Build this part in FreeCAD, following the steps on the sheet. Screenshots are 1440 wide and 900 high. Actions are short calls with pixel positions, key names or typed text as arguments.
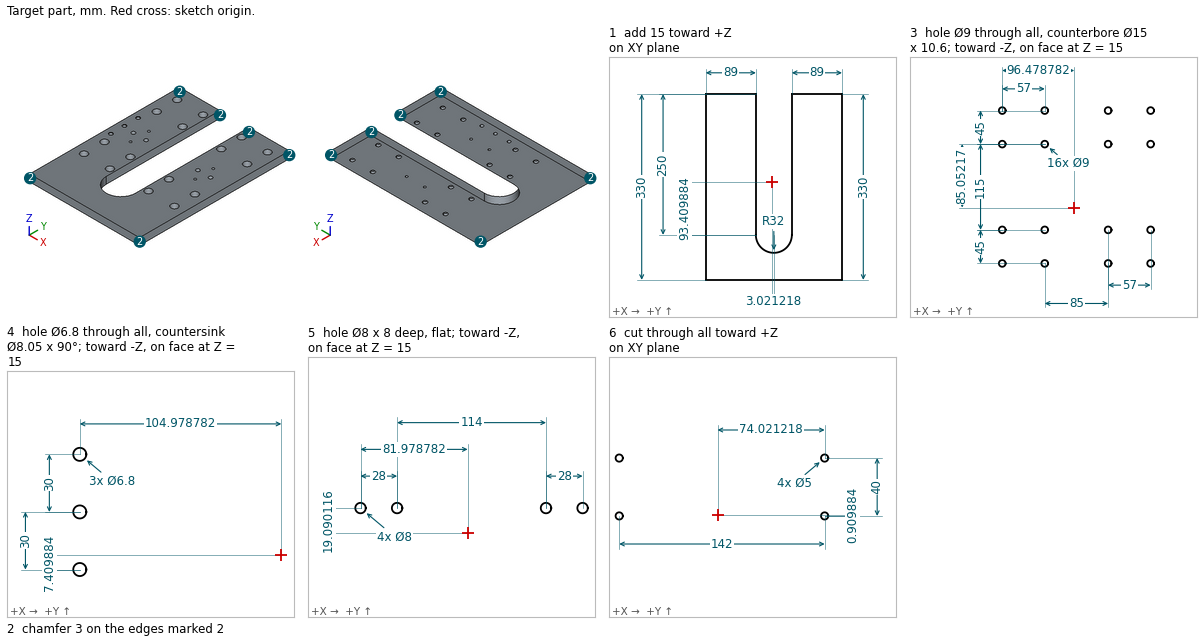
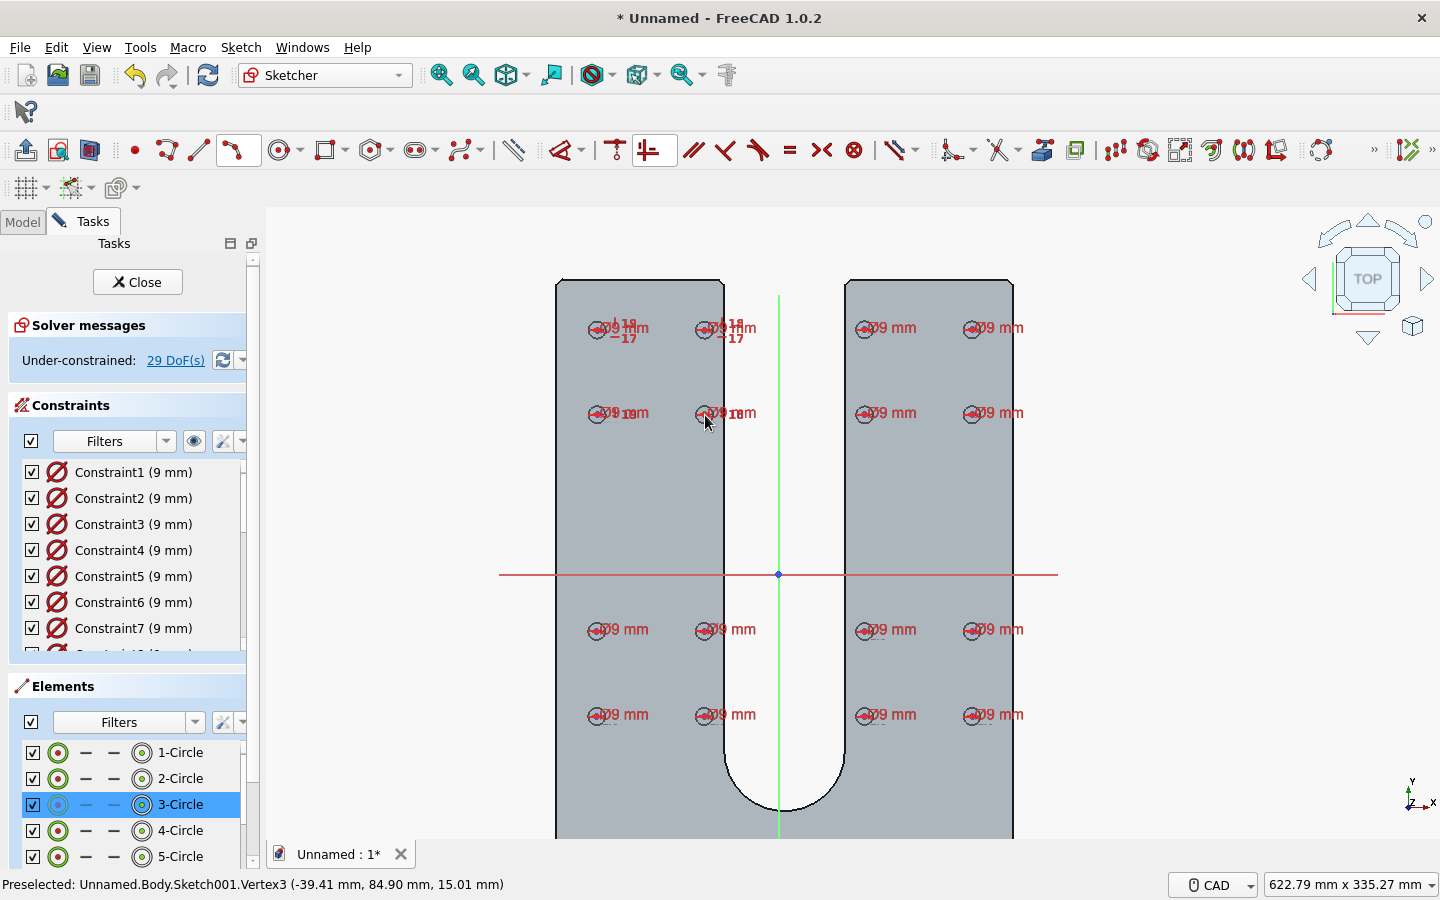
click(597, 415)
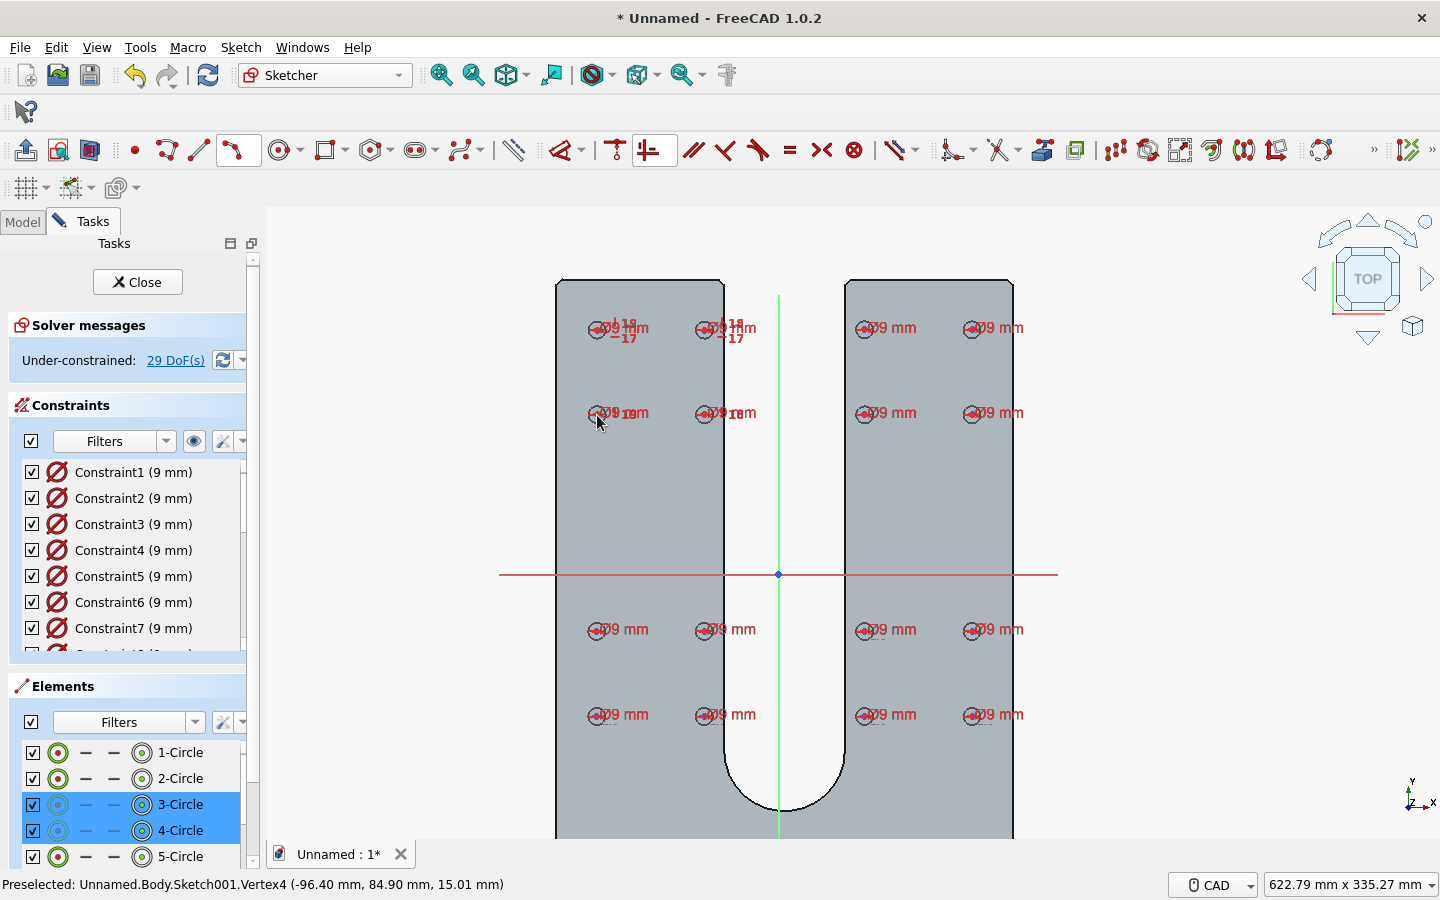
key(h)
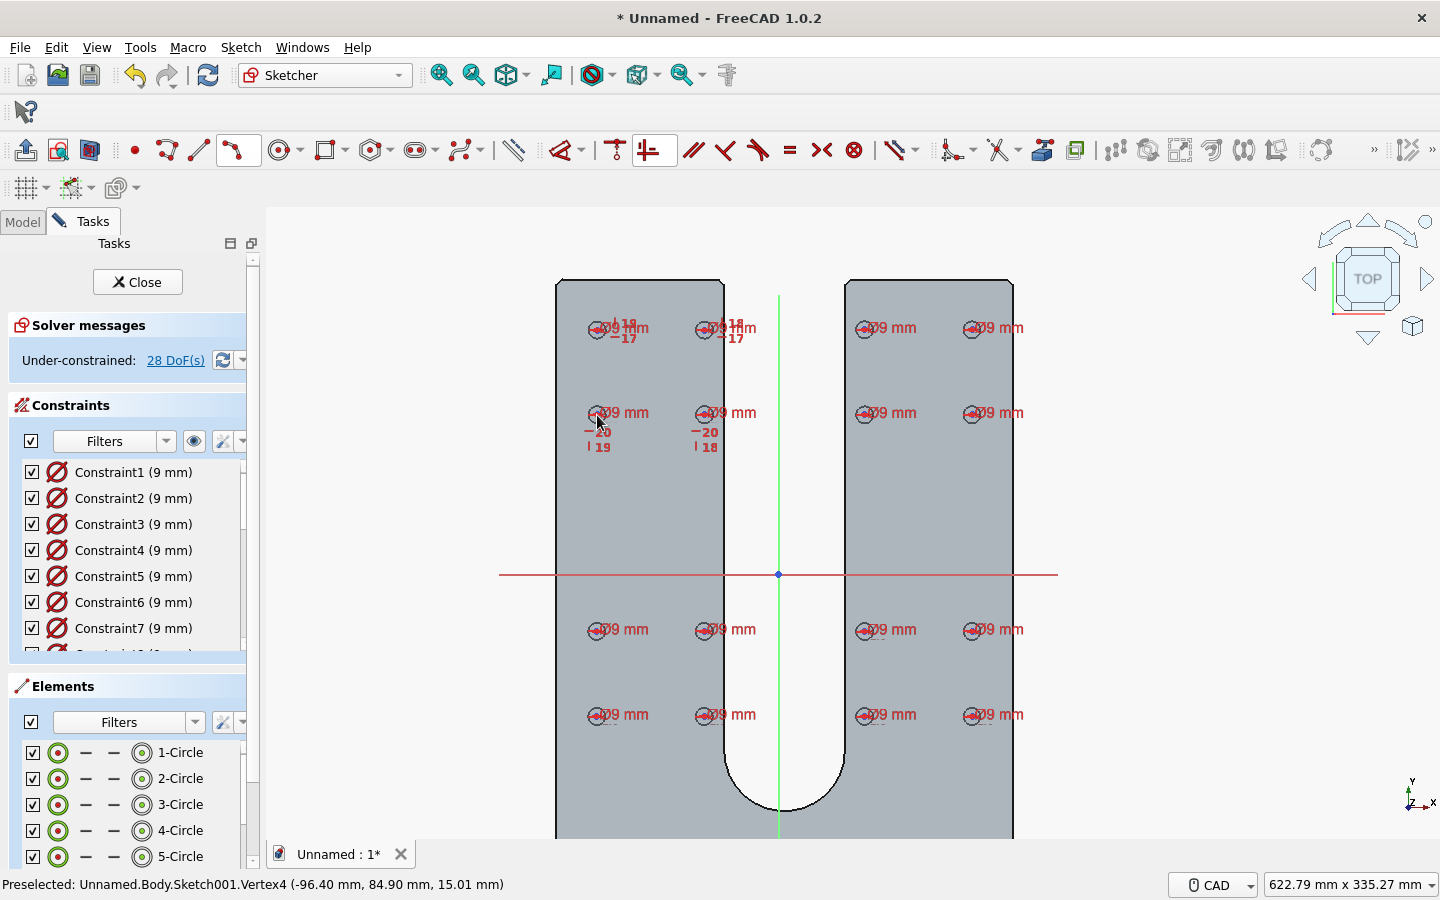
click(597, 415)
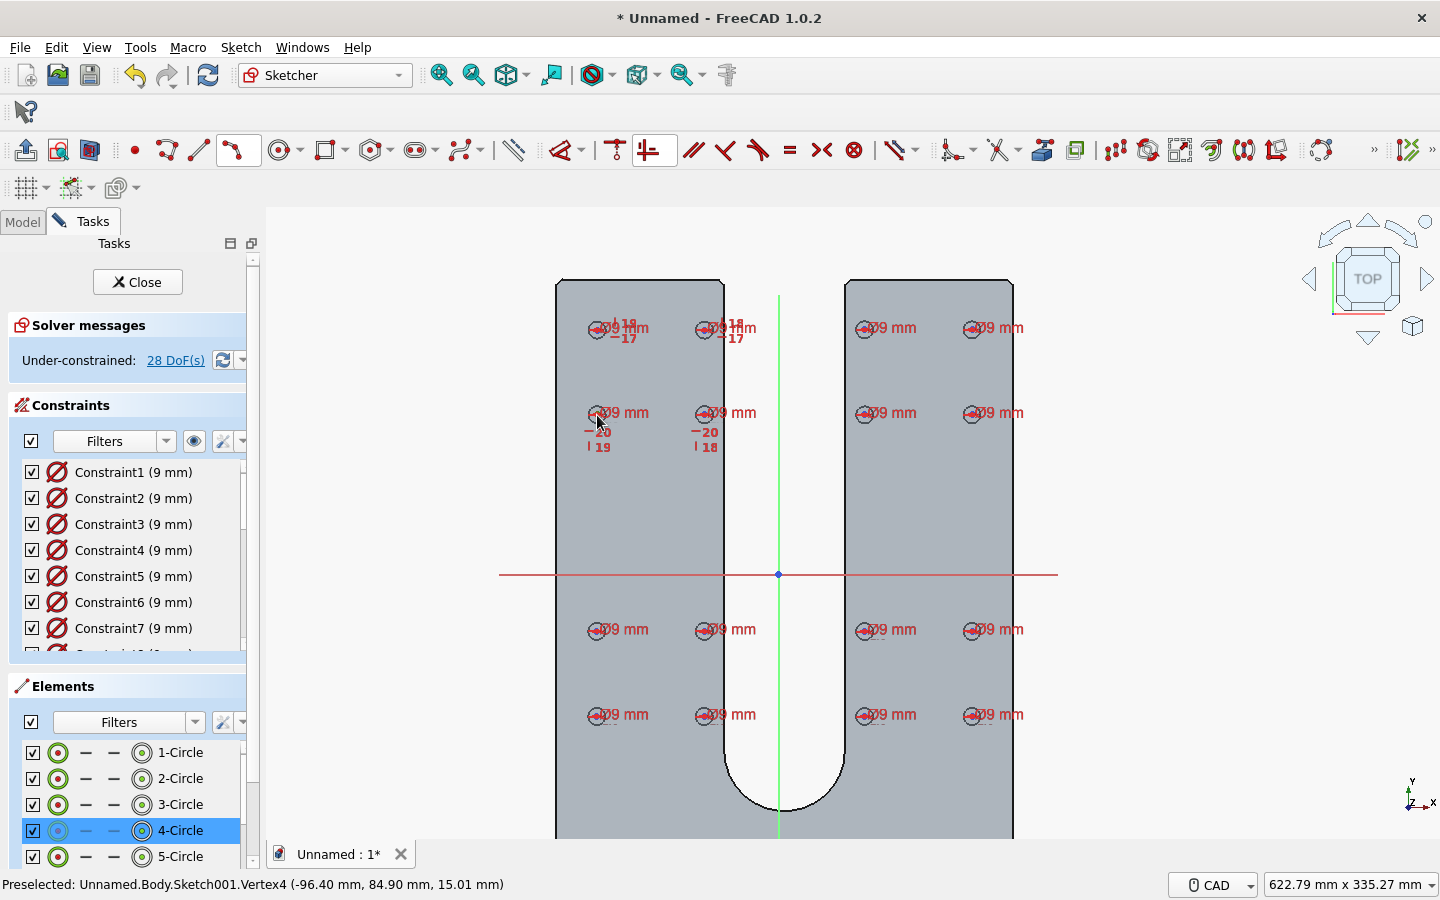
click(597, 631)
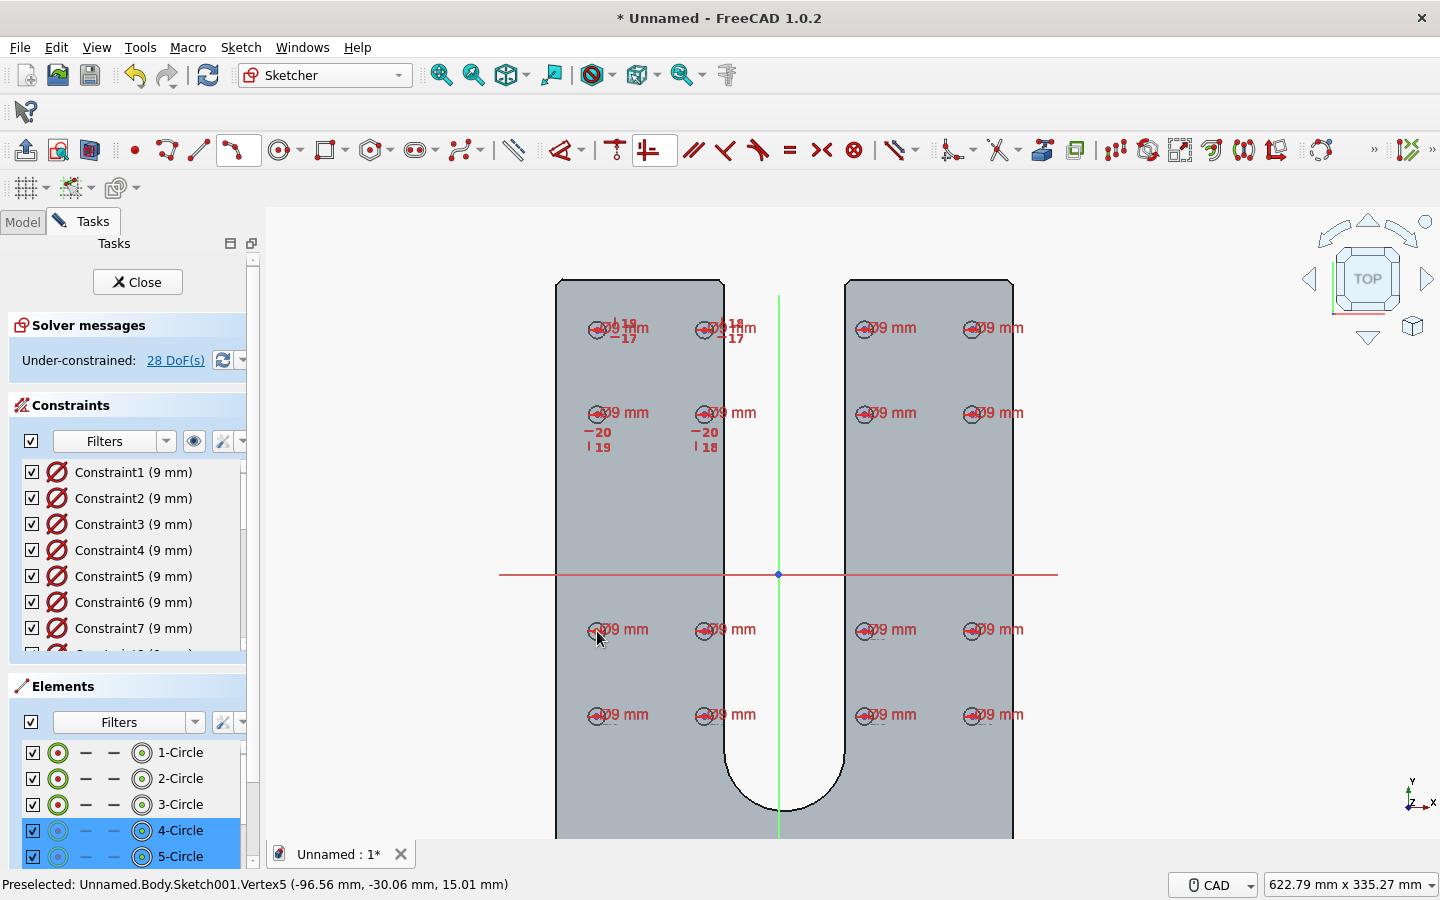
key(v)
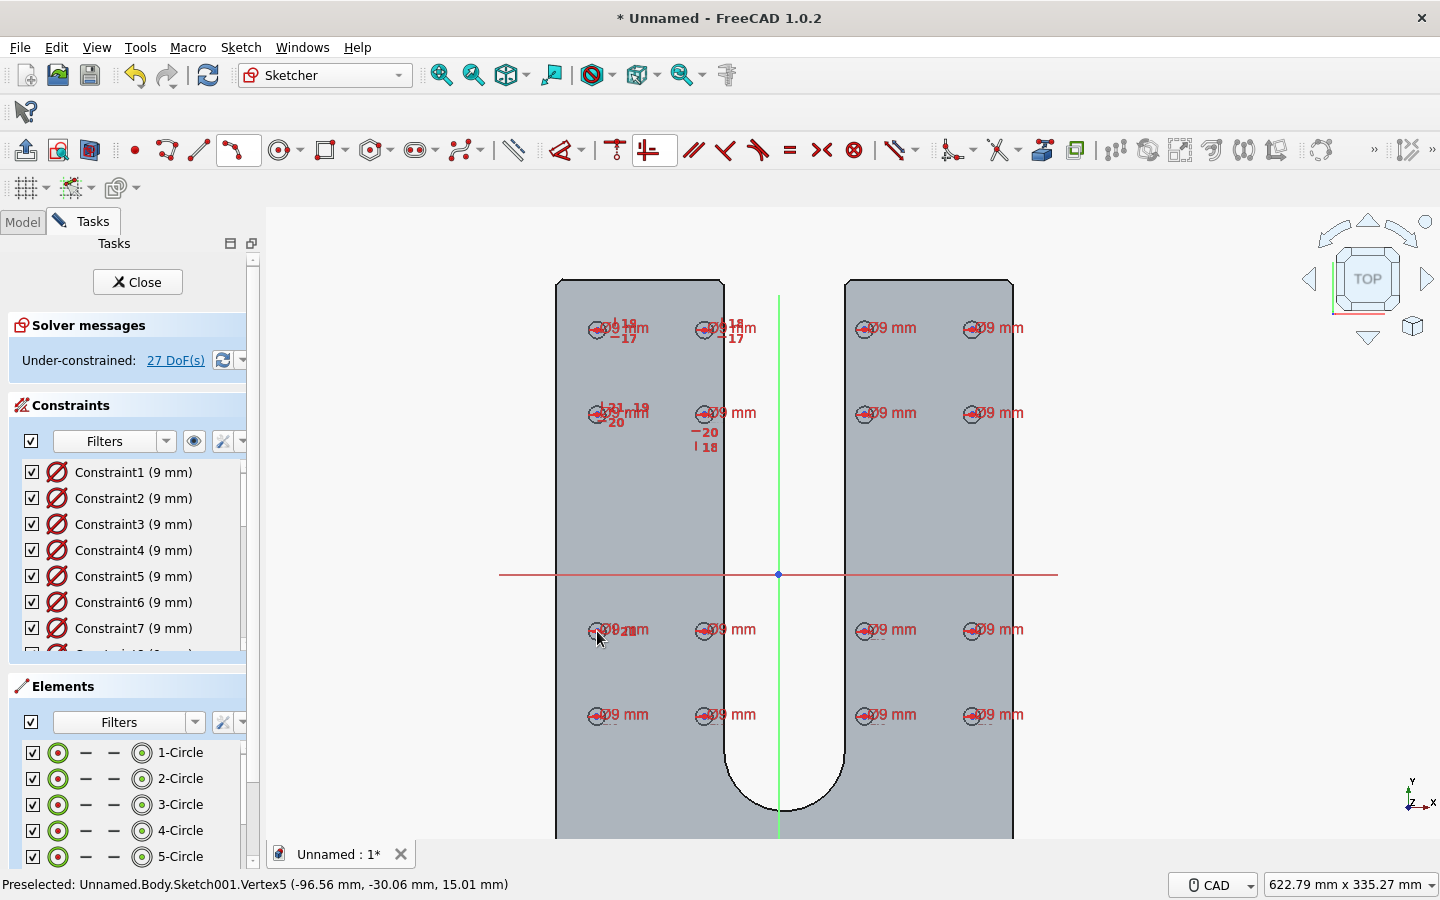
click(705, 415)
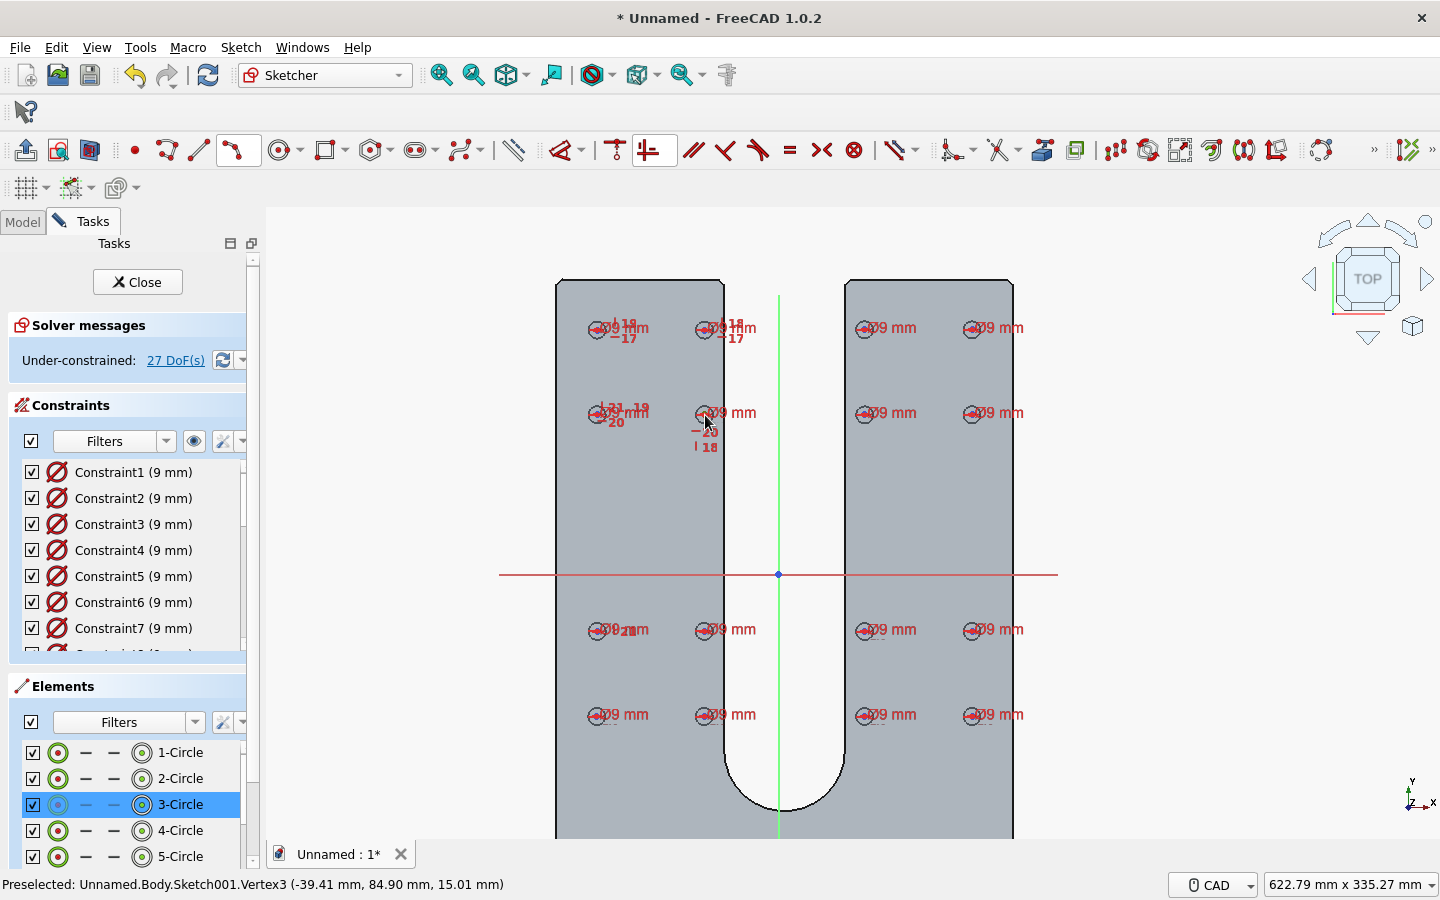
click(704, 631)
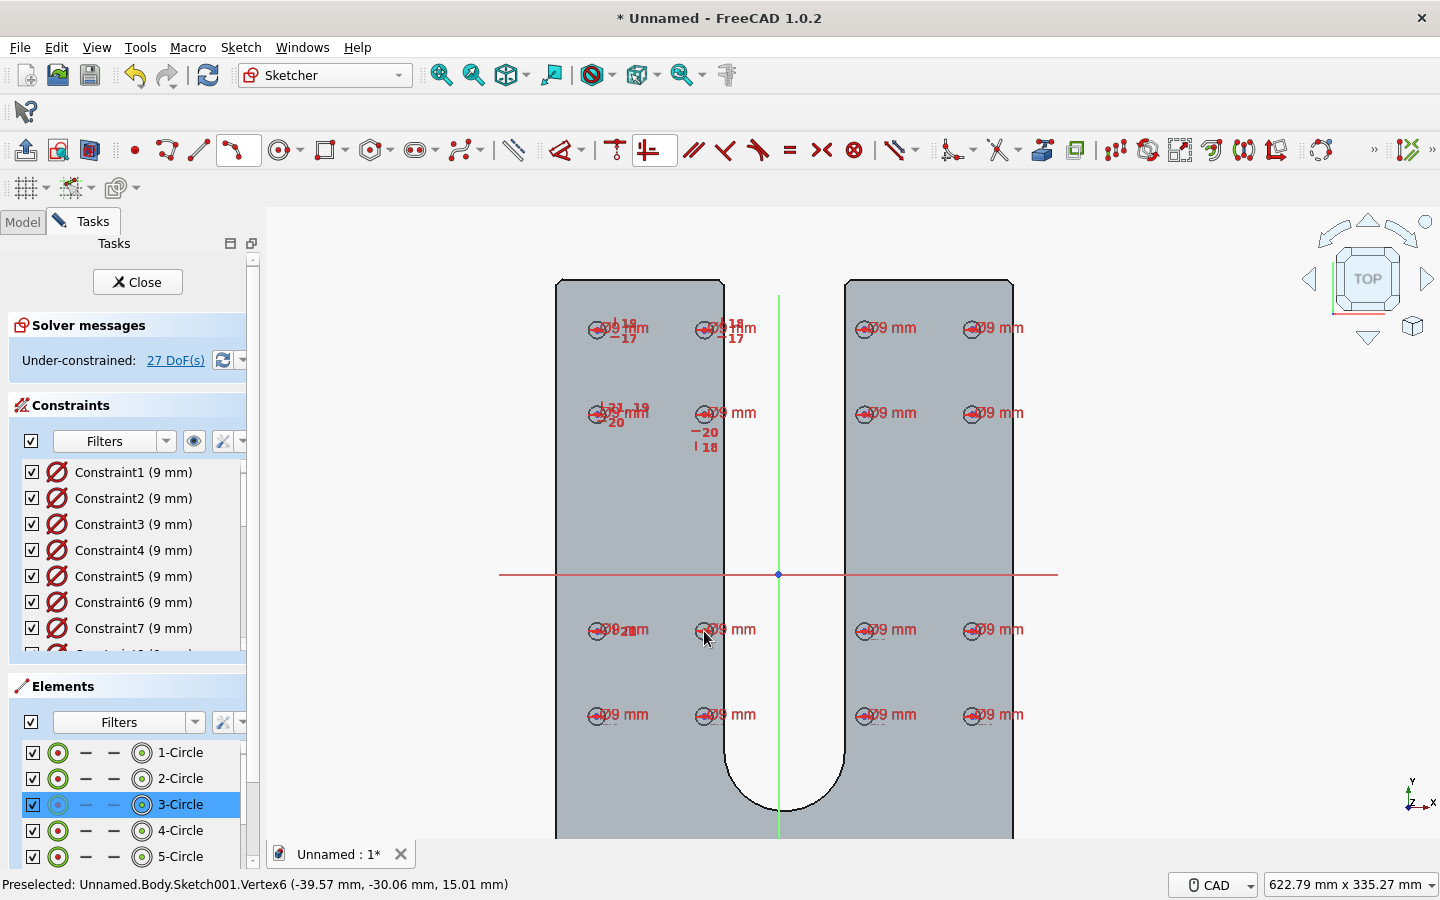
click(672, 150)